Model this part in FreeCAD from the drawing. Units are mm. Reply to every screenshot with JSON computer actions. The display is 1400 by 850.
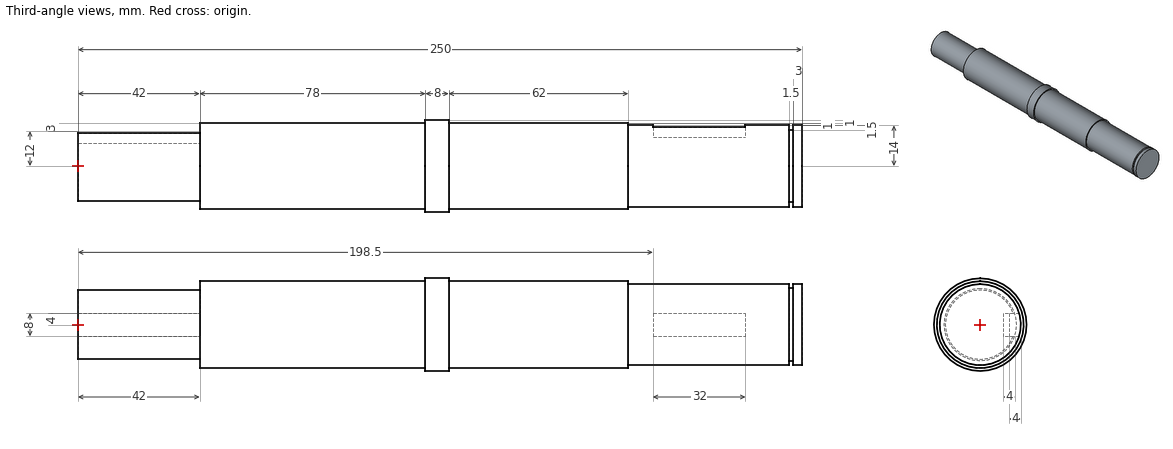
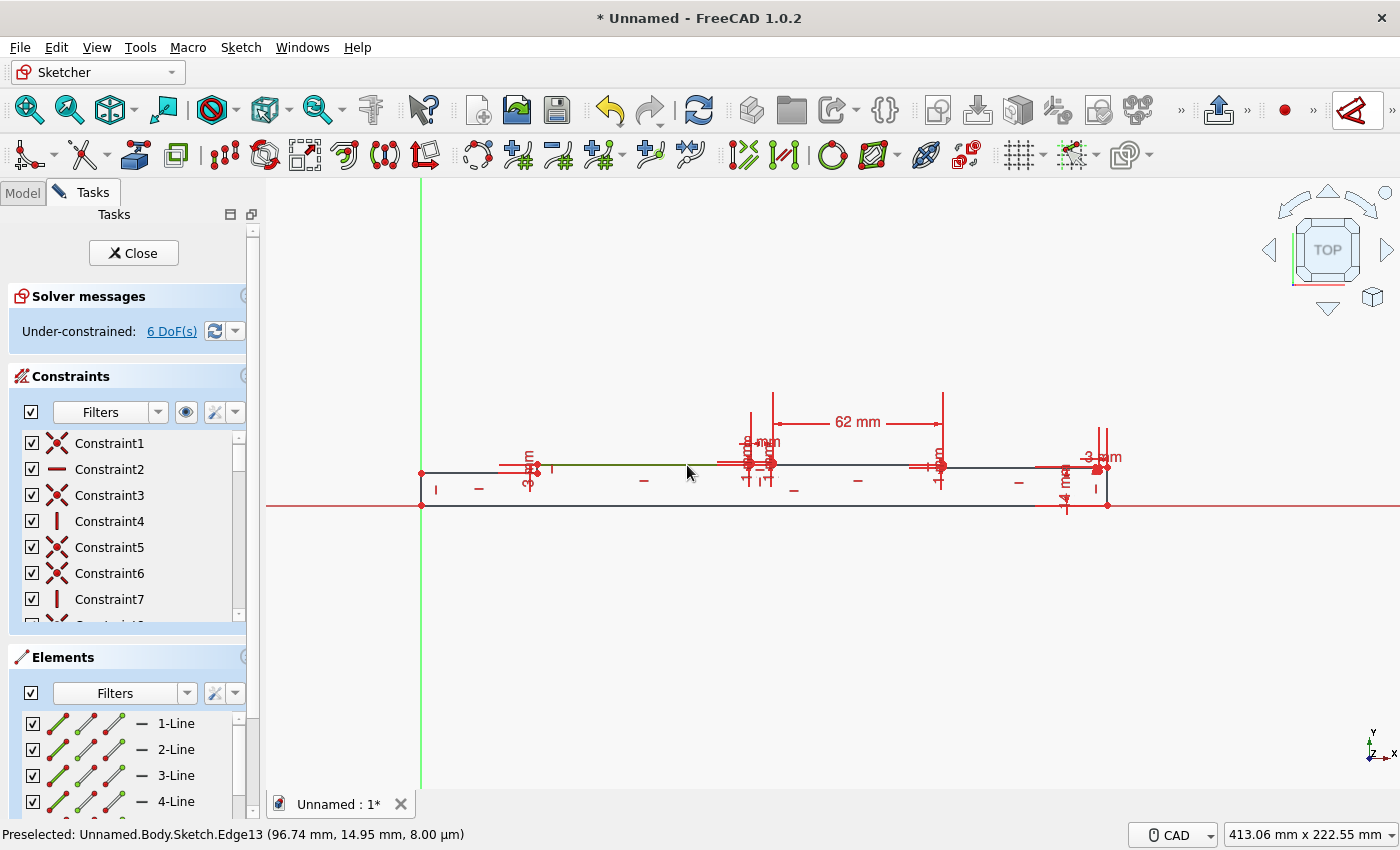
{"action": "left_click", "coordinate": [1378, 110]}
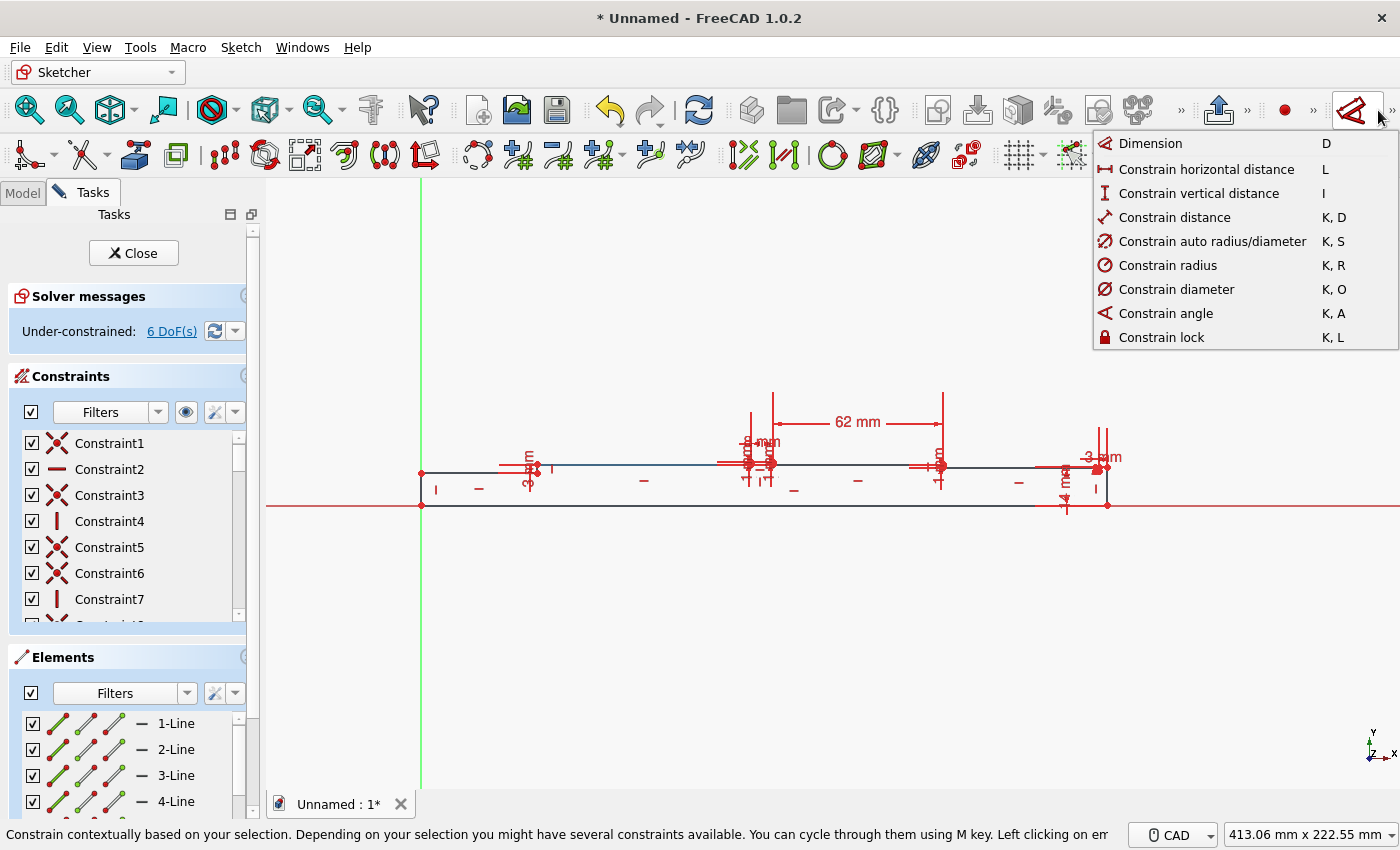
{"action": "left_click", "coordinate": [1246, 169]}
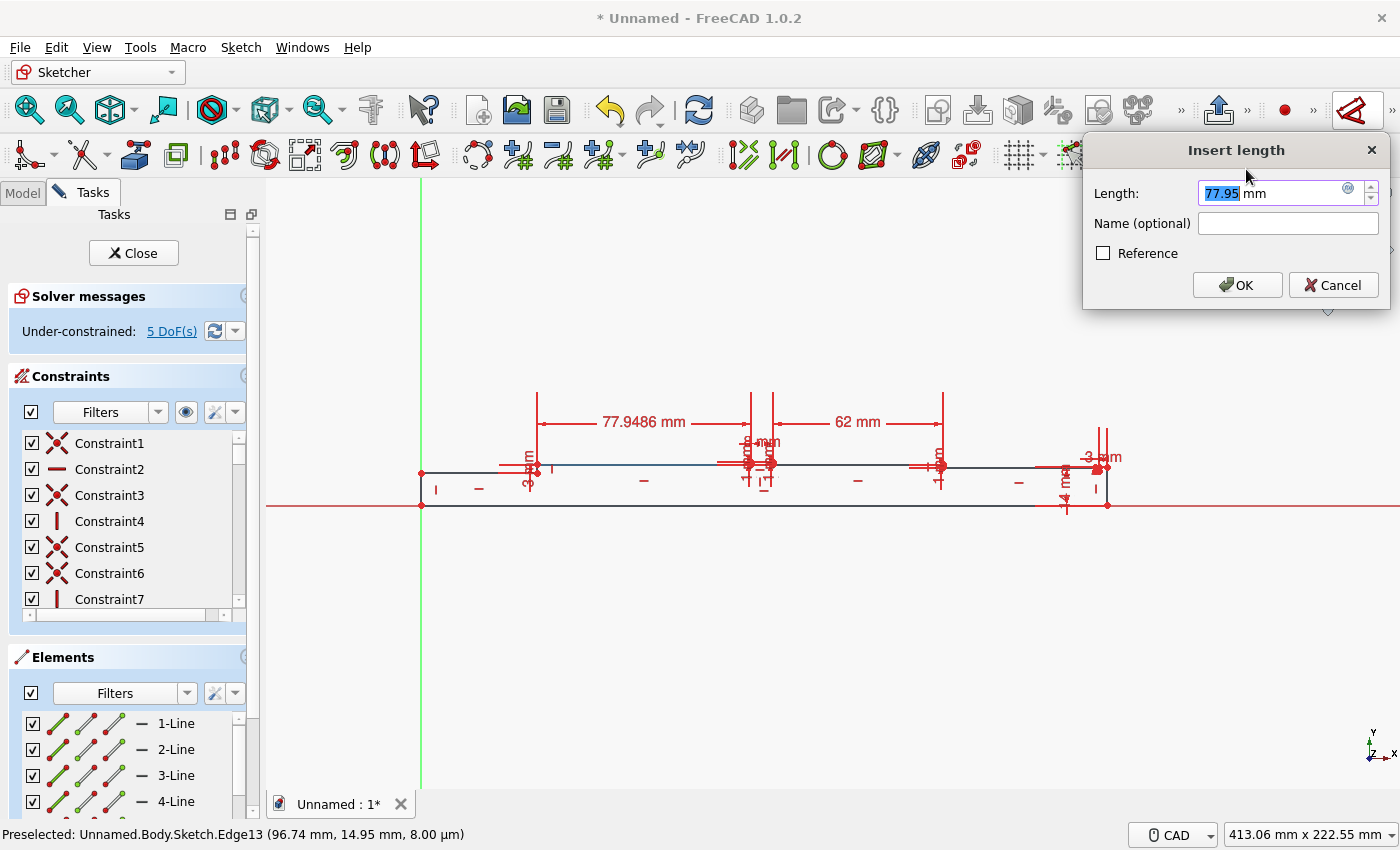
{"action": "type", "text": "78"}
{"action": "key", "text": "Return"}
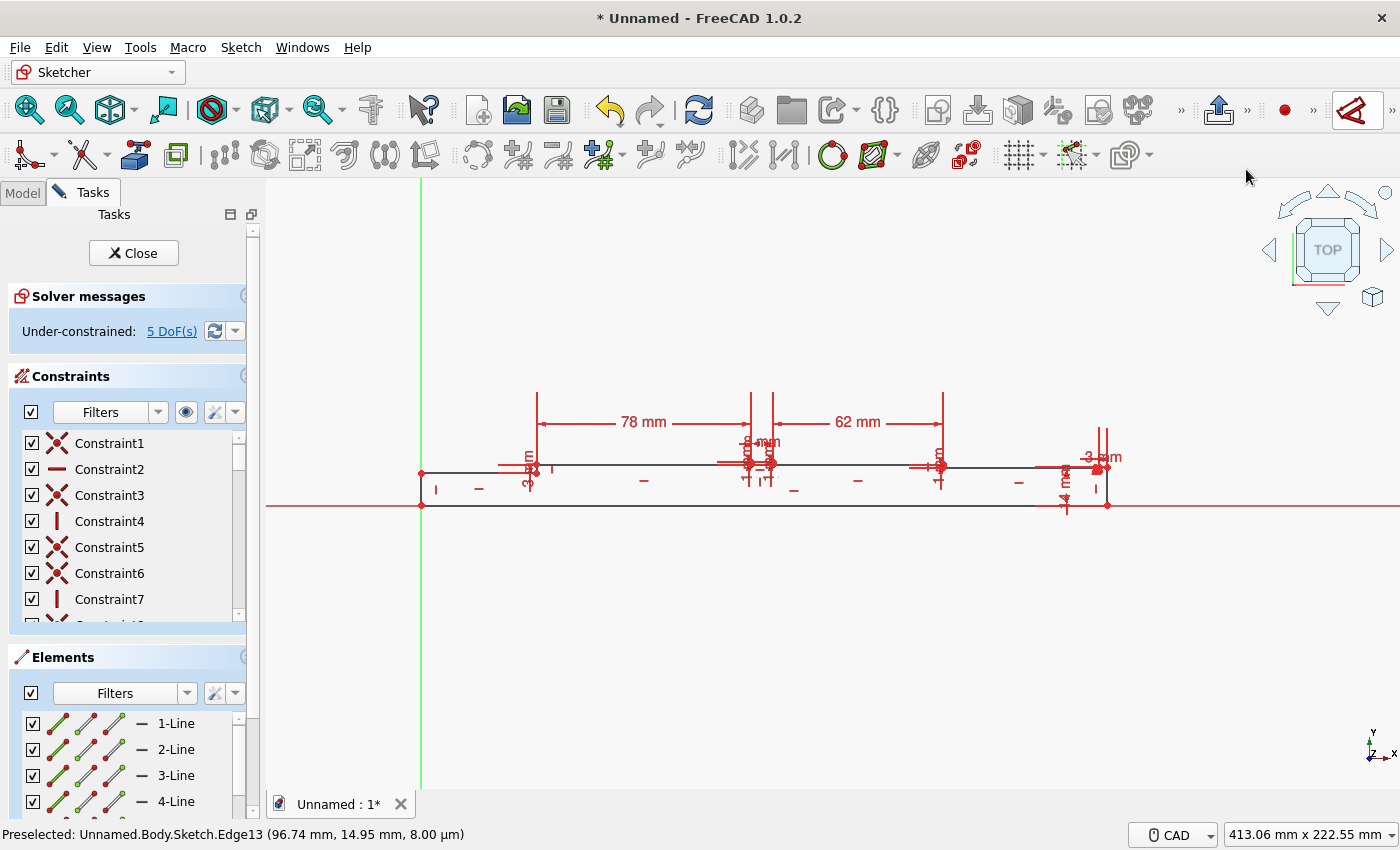
{"action": "left_click", "coordinate": [502, 473]}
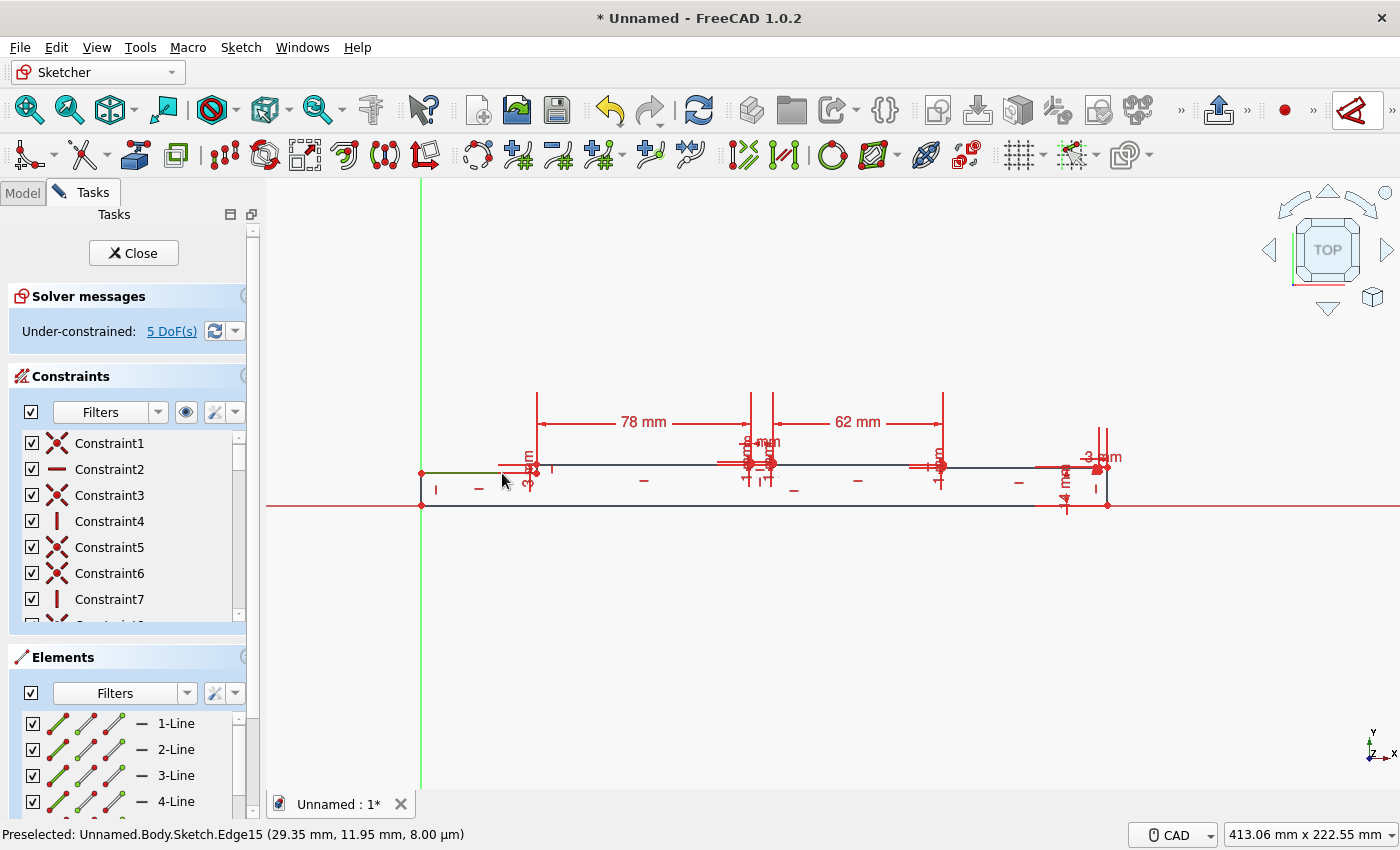
{"action": "key", "text": "l"}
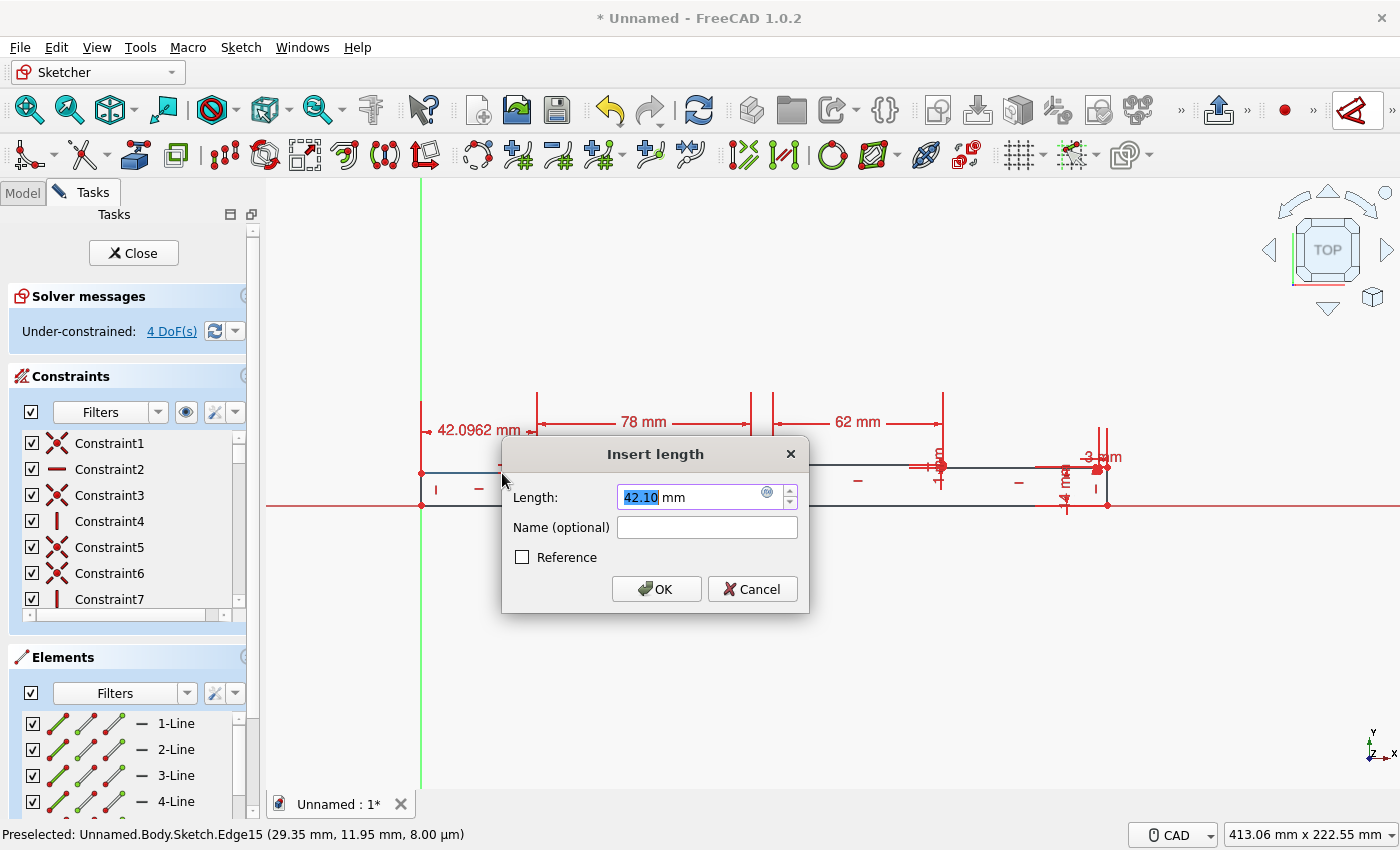
{"action": "type", "text": "42"}
{"action": "key", "text": "Return"}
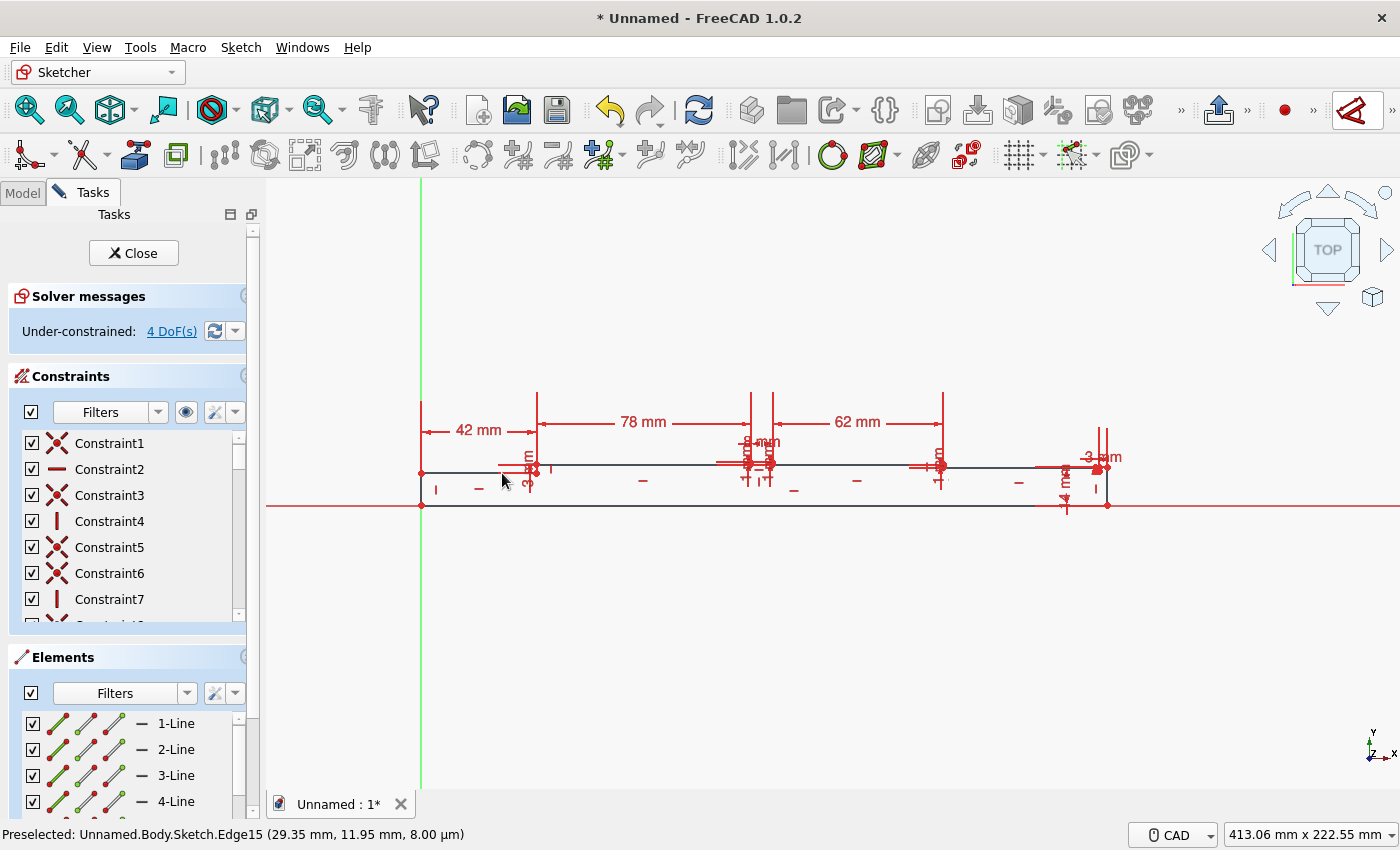
{"action": "scroll", "coordinate": [421, 483], "scroll_direction": "up", "scroll_amount": 2}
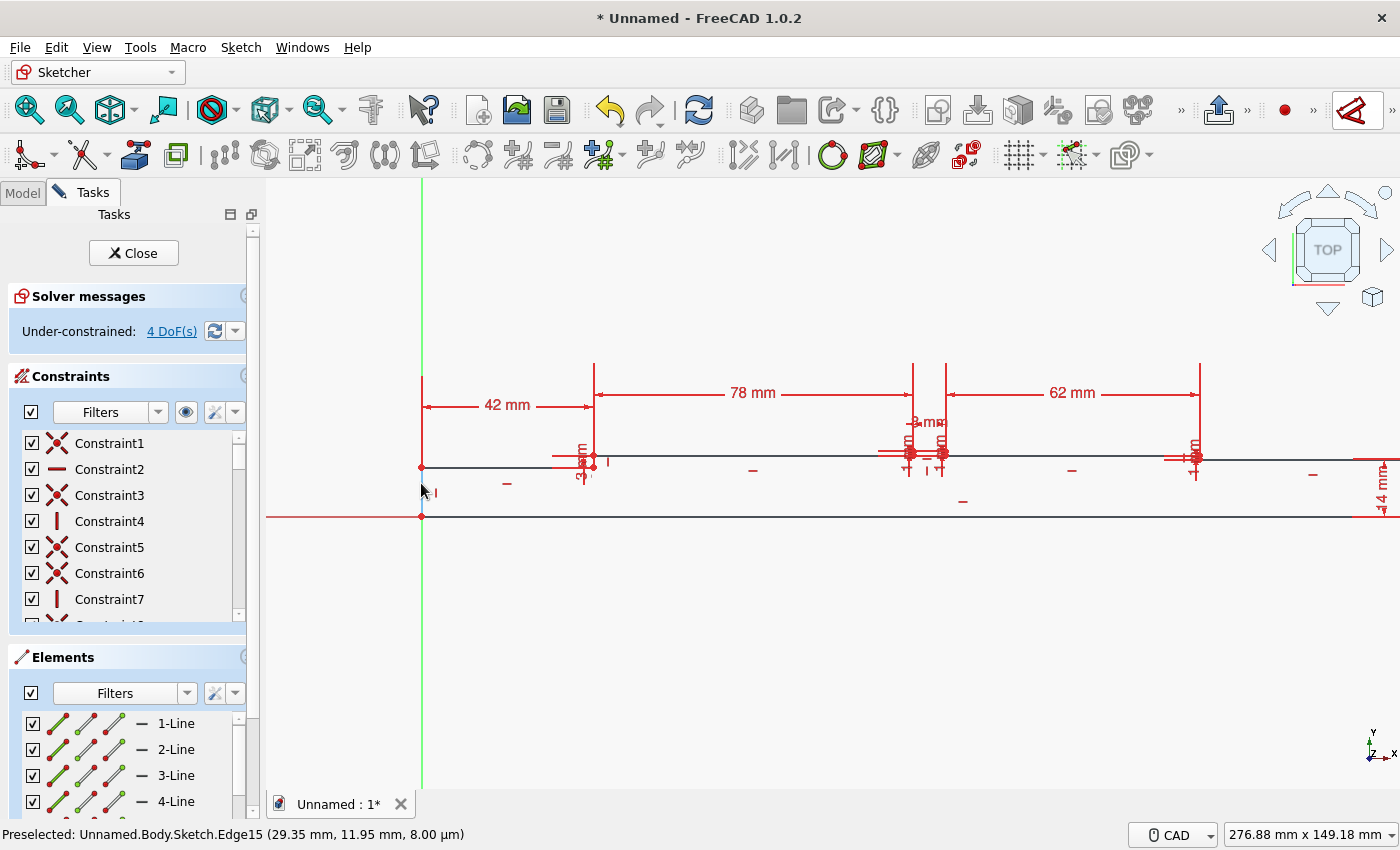
{"action": "left_click", "coordinate": [422, 483]}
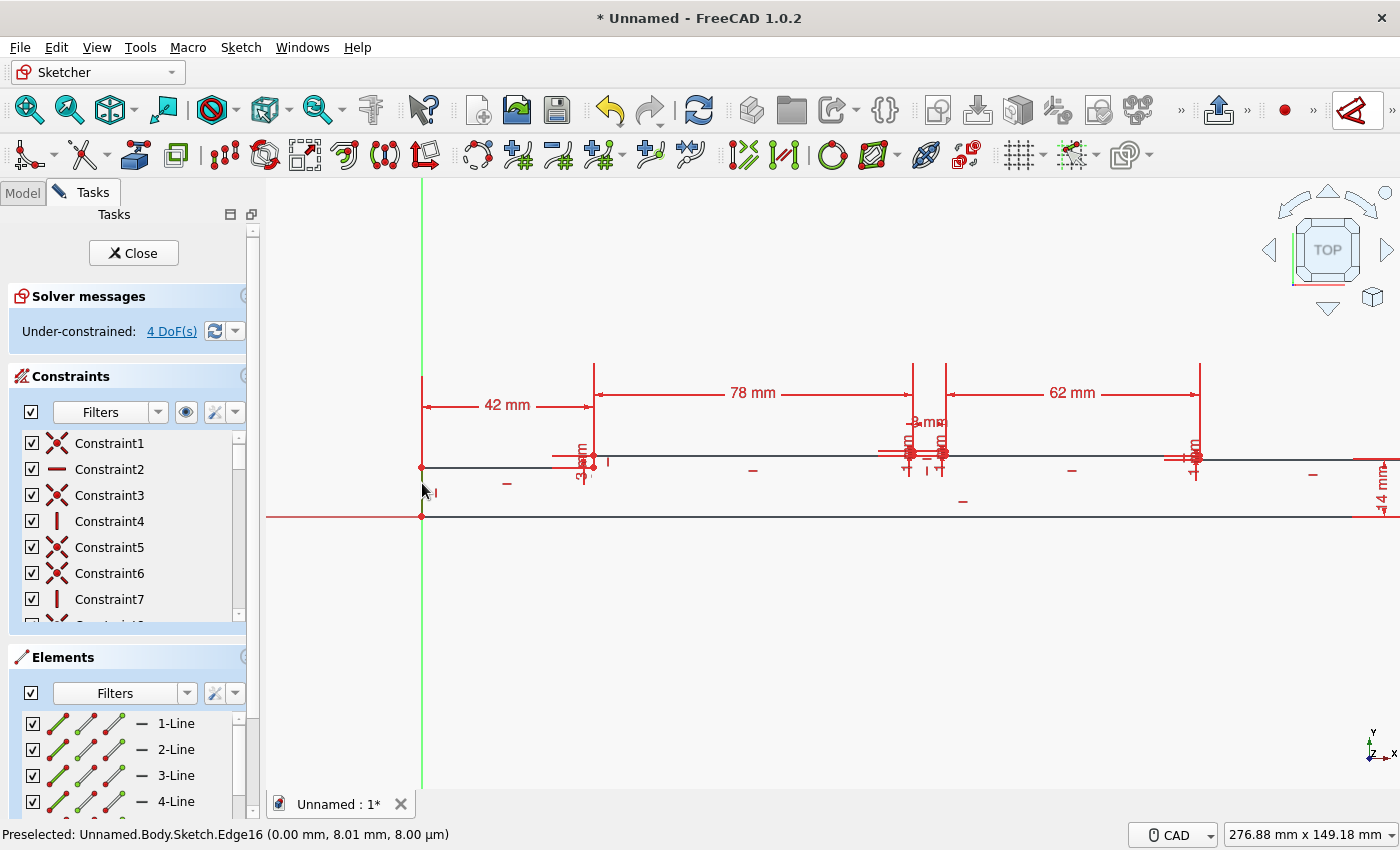
{"action": "key", "text": "i"}